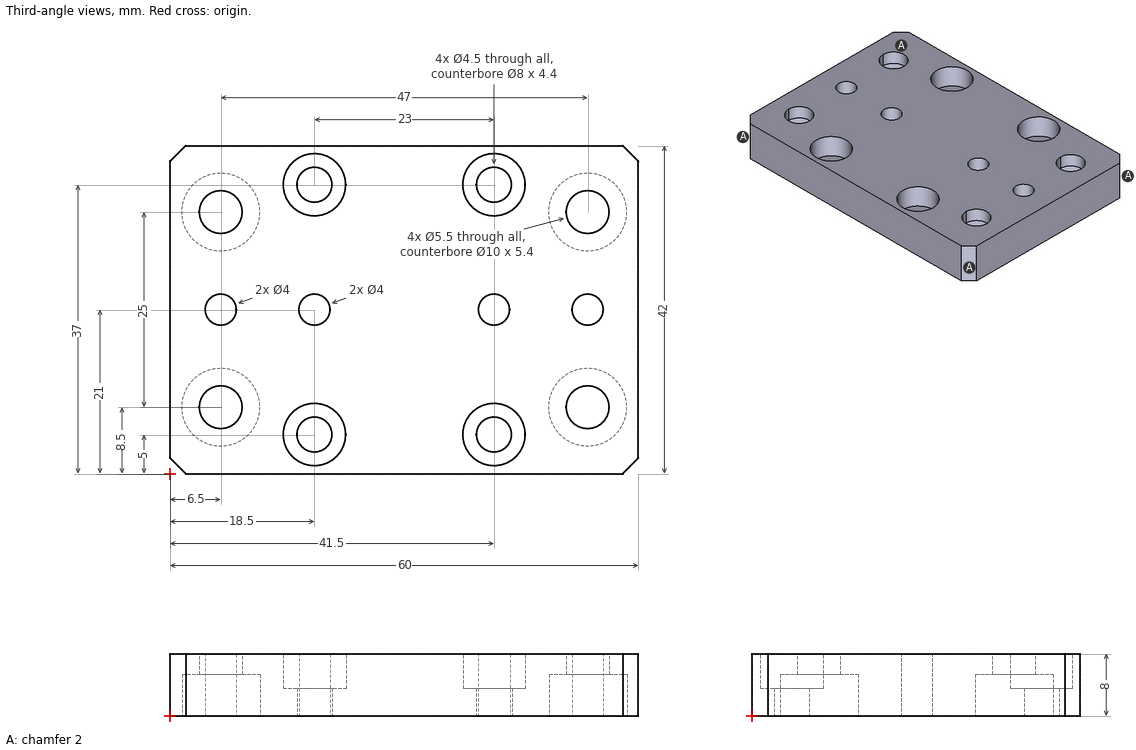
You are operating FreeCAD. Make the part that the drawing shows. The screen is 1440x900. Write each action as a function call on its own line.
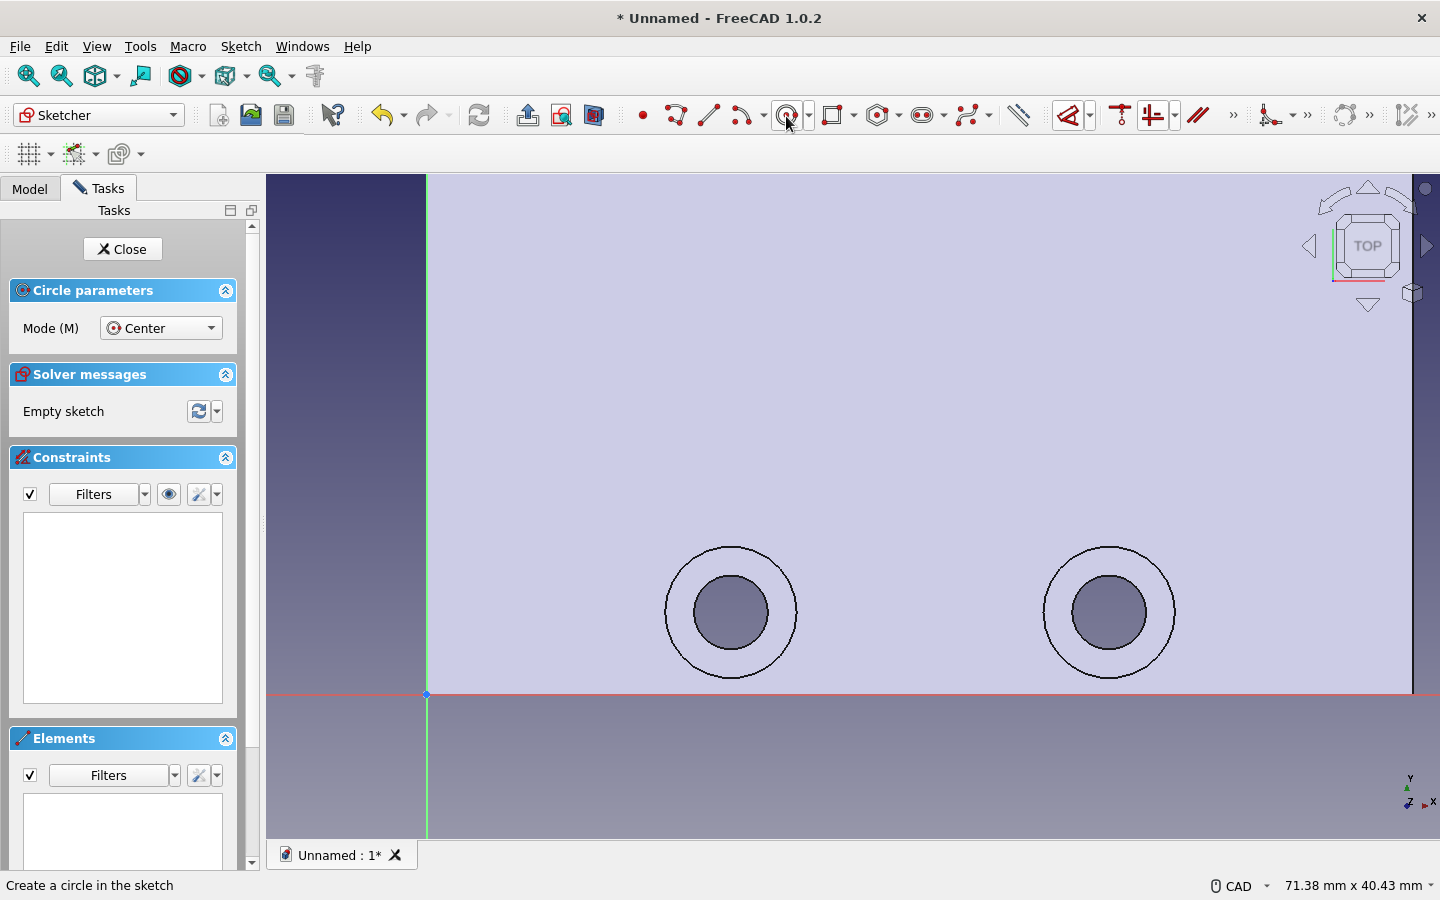
click(731, 349)
click(754, 326)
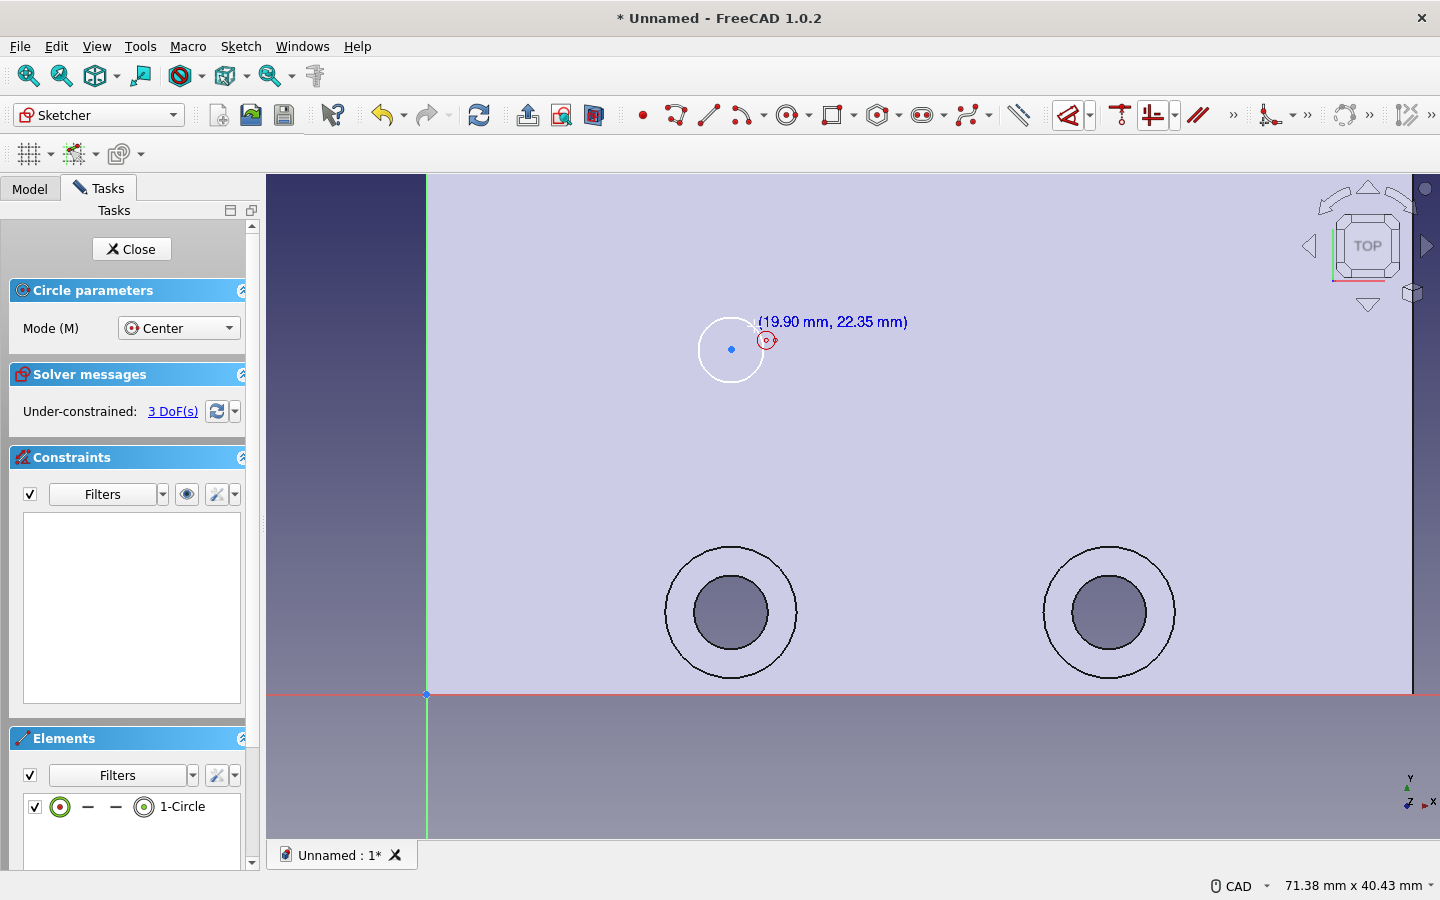
click(1109, 349)
click(1132, 326)
key(Escape)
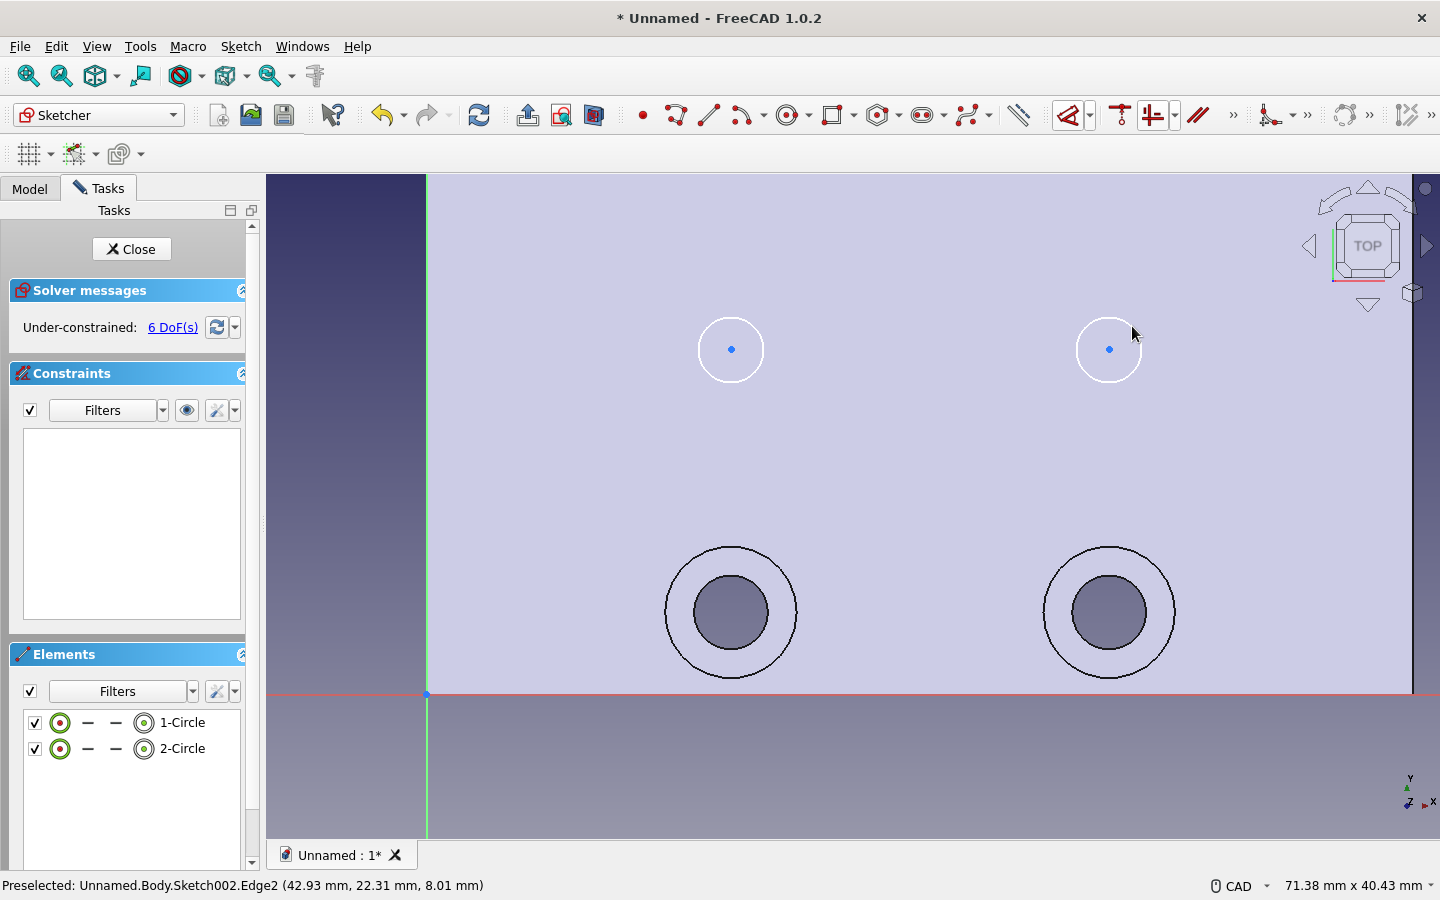
click(754, 327)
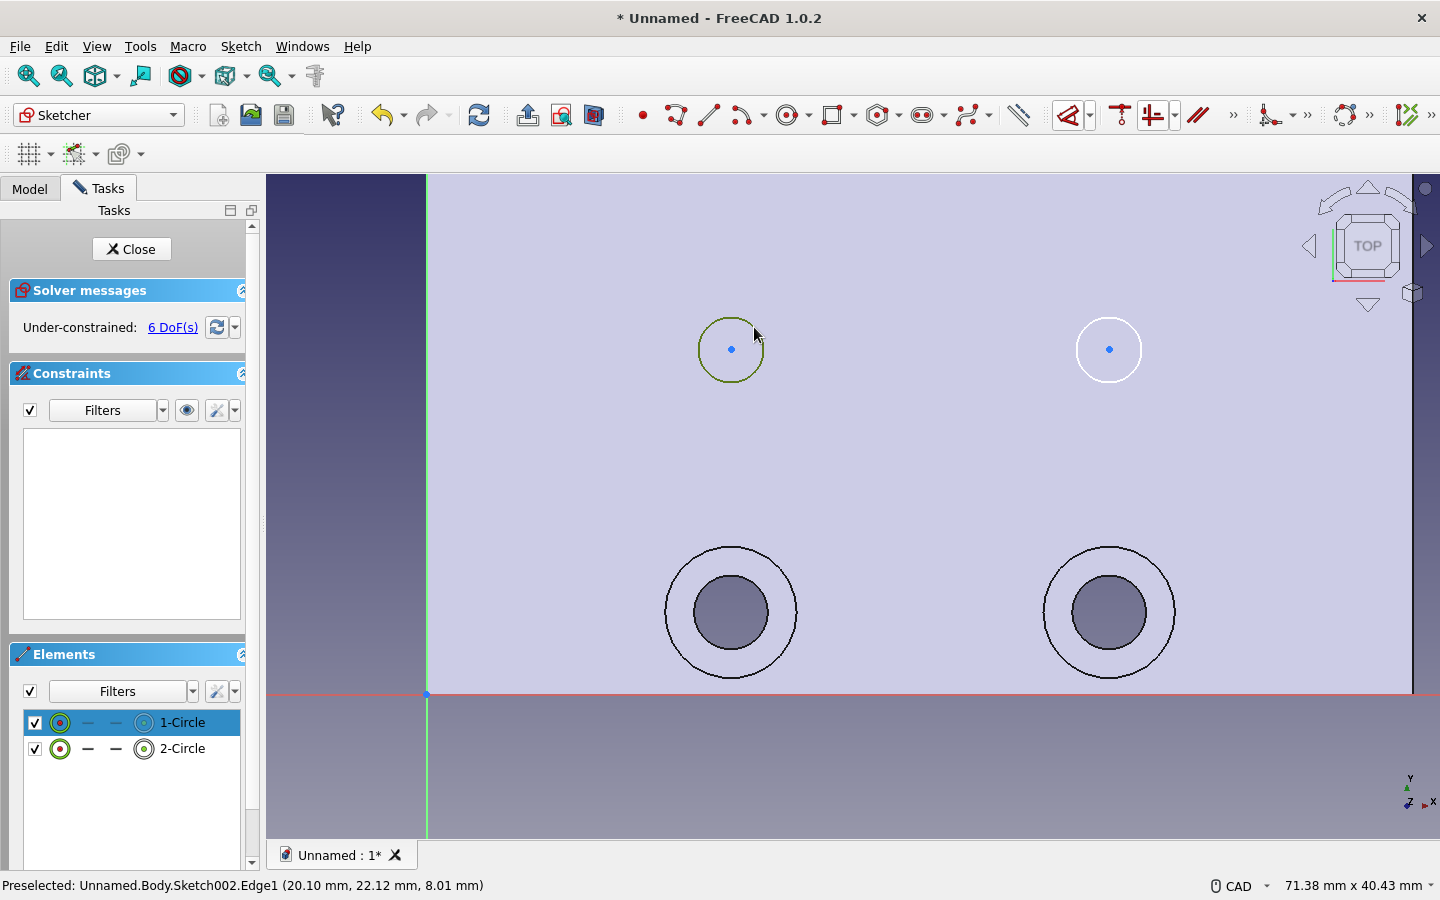
click(1132, 327)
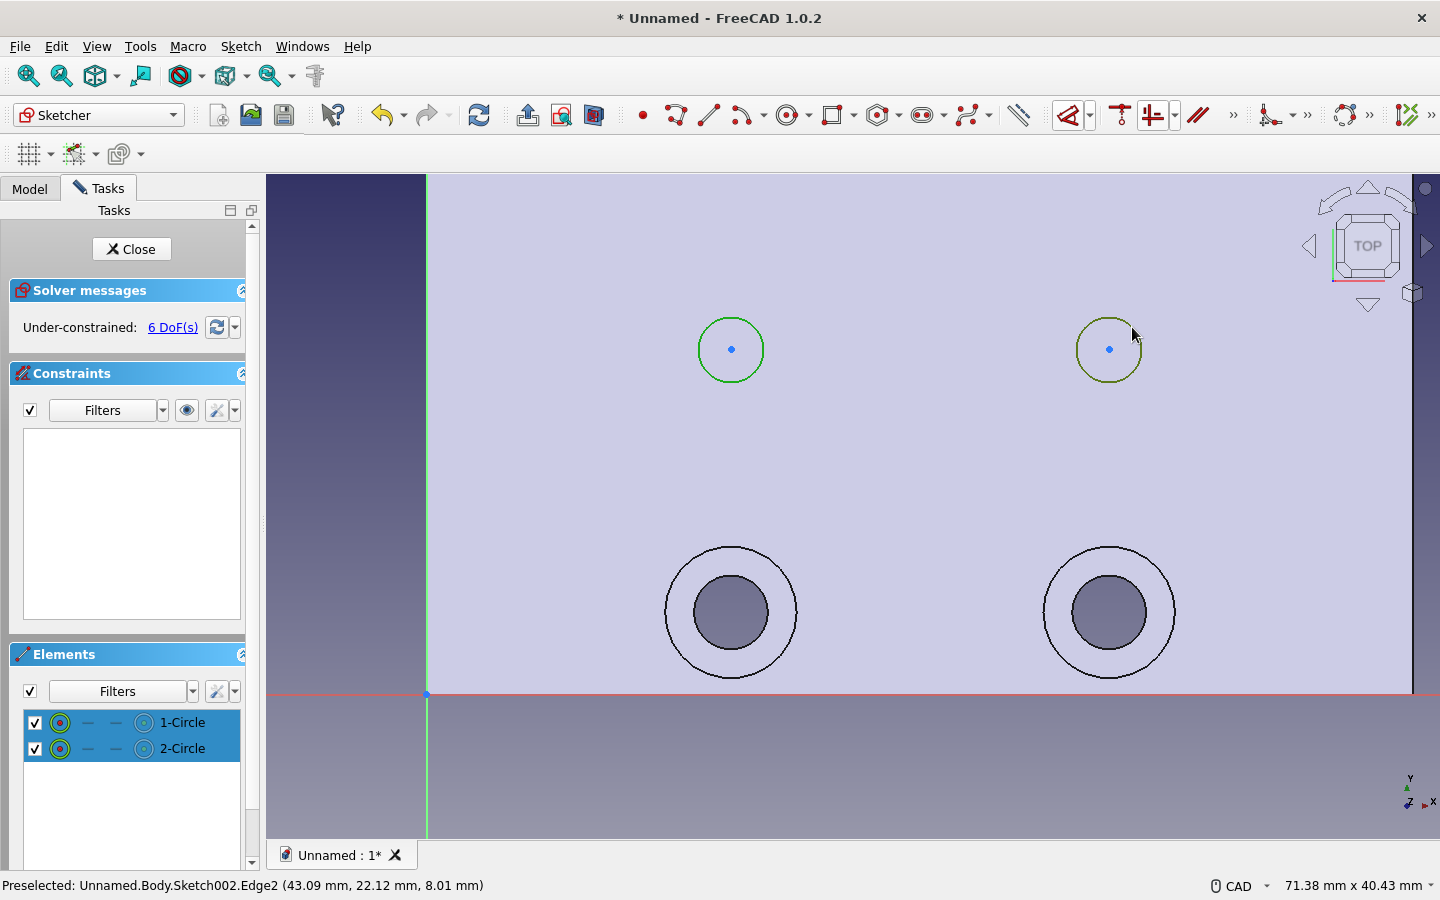
key(e)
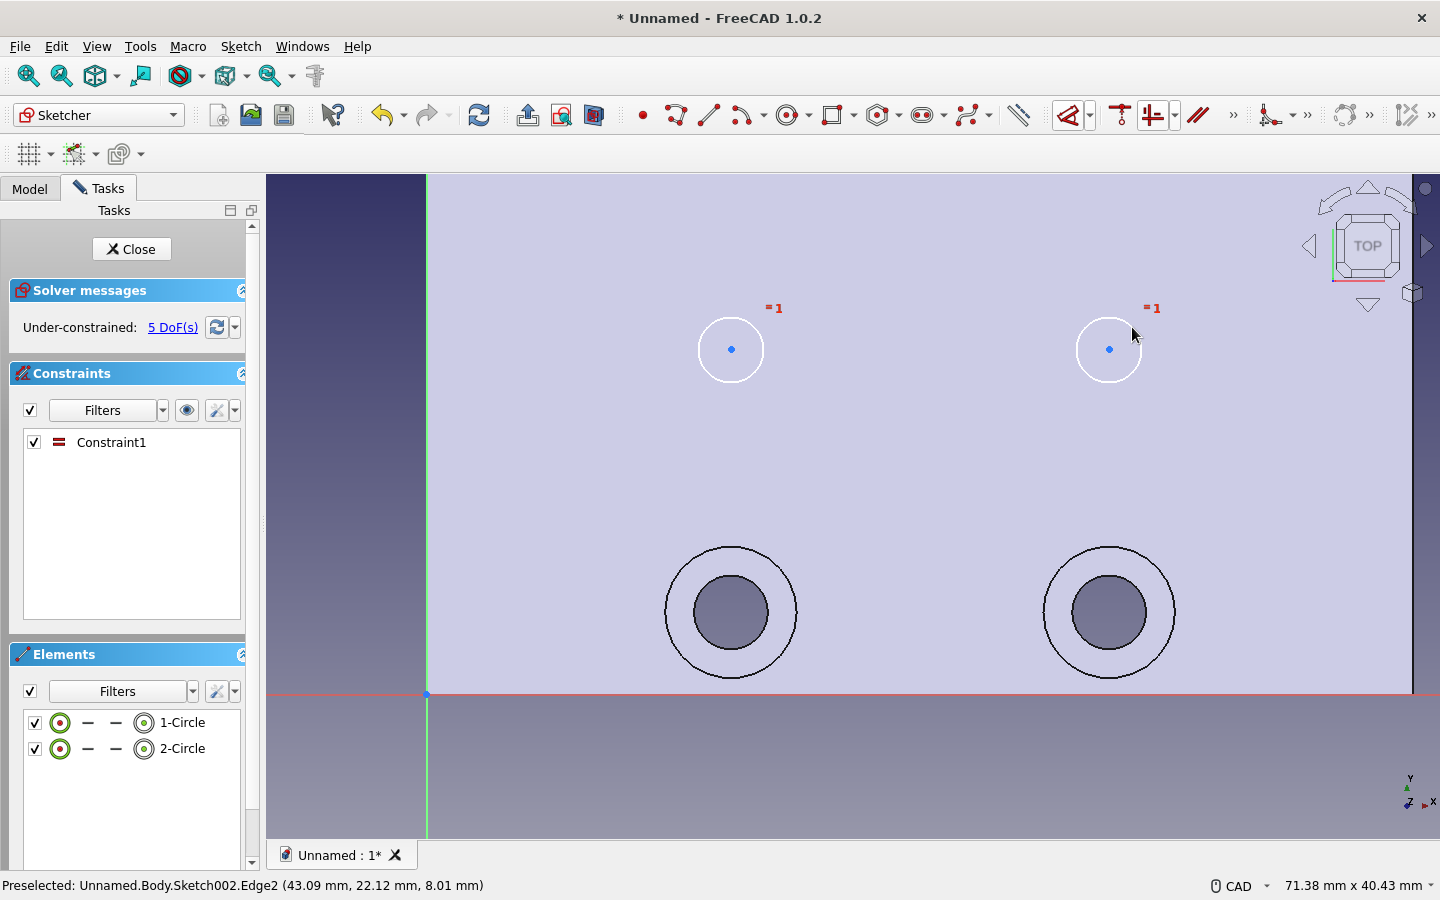
click(731, 350)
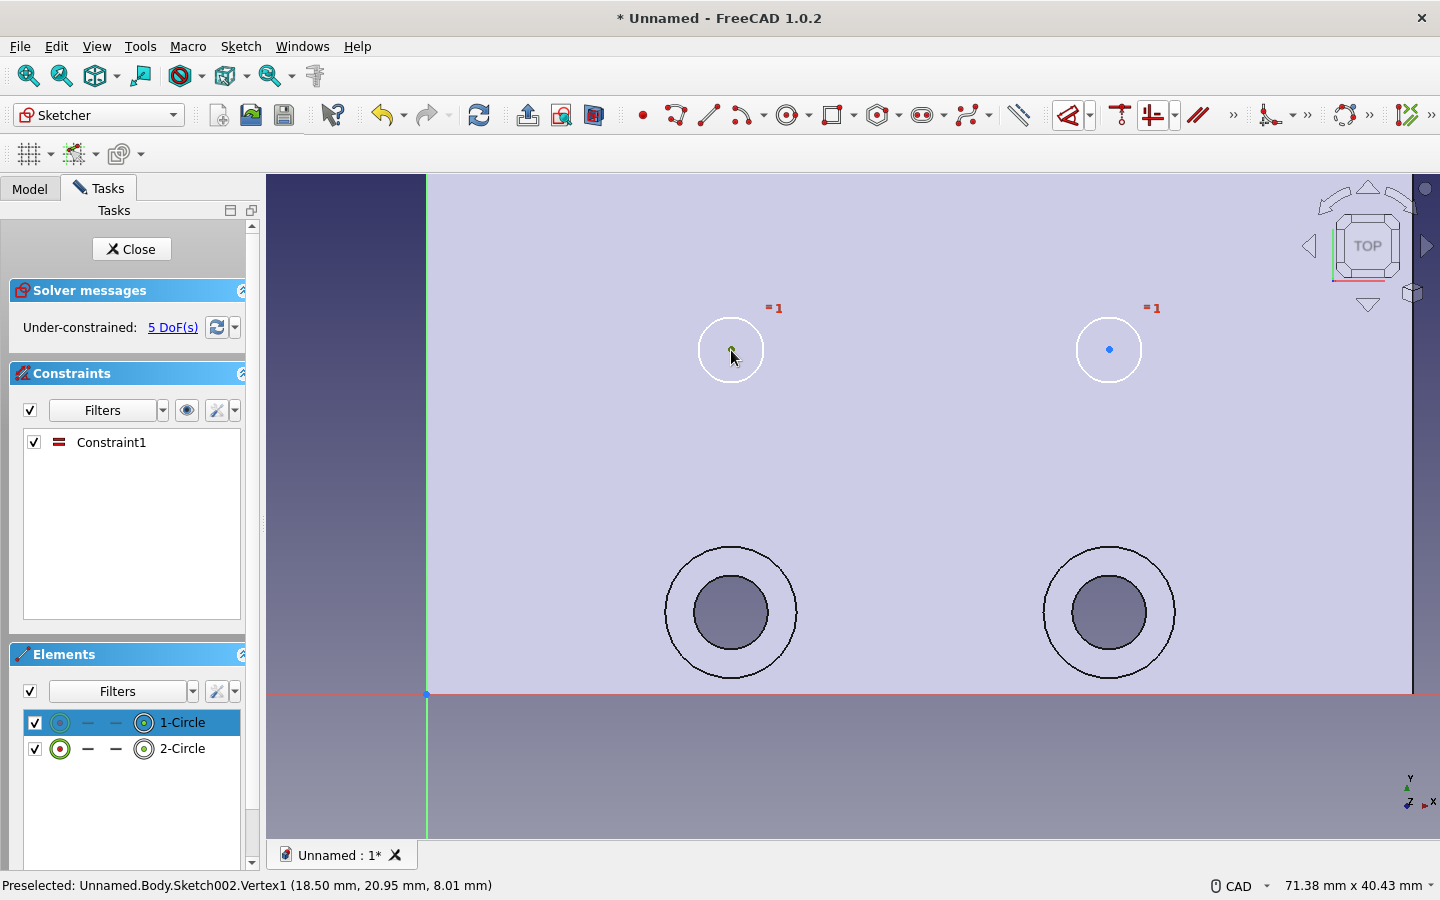
click(1109, 350)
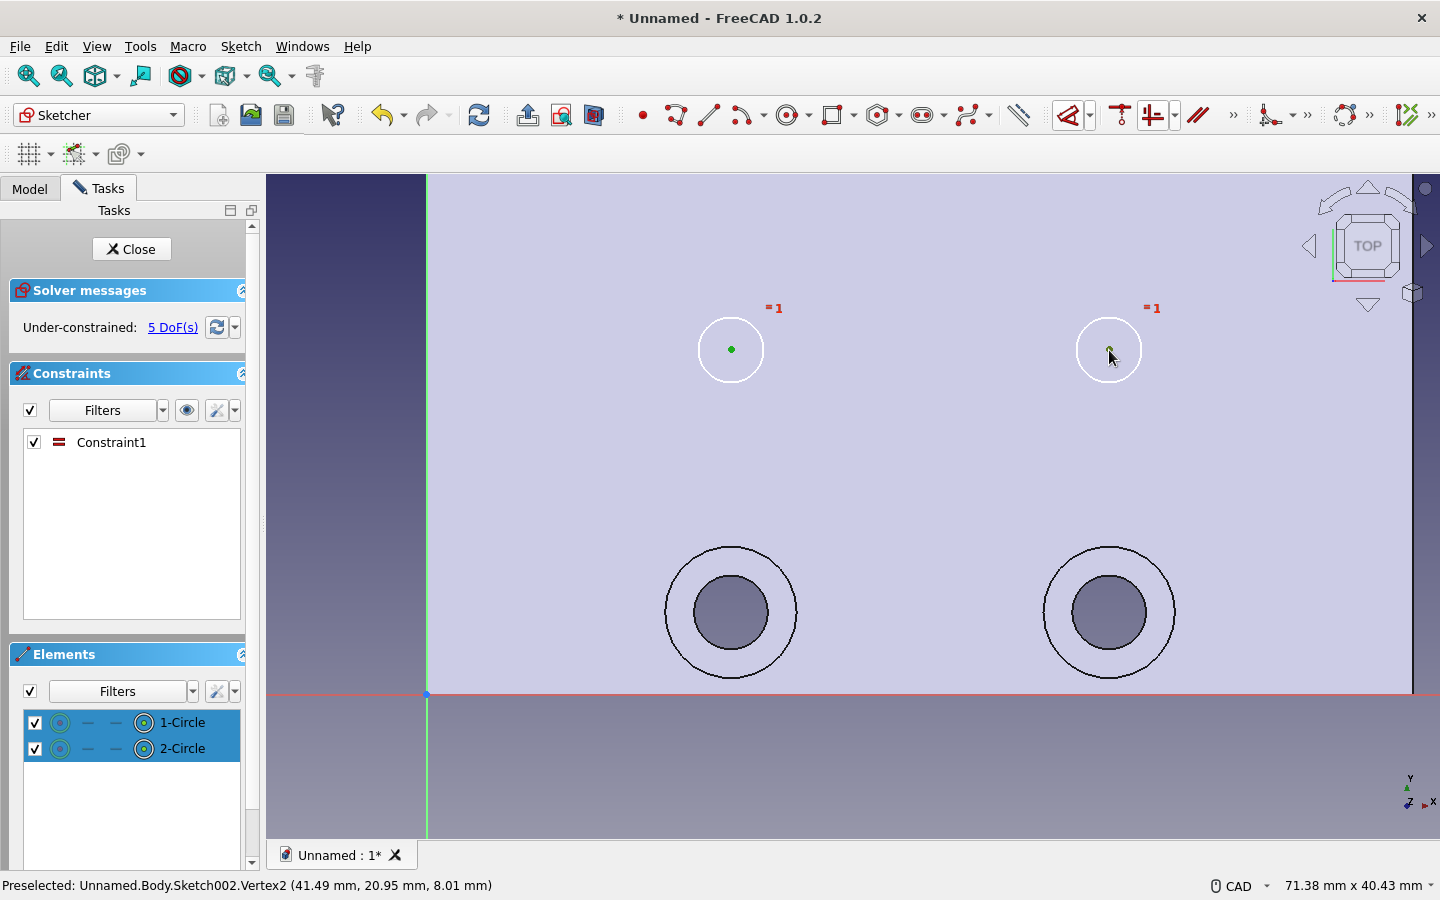
click(1174, 116)